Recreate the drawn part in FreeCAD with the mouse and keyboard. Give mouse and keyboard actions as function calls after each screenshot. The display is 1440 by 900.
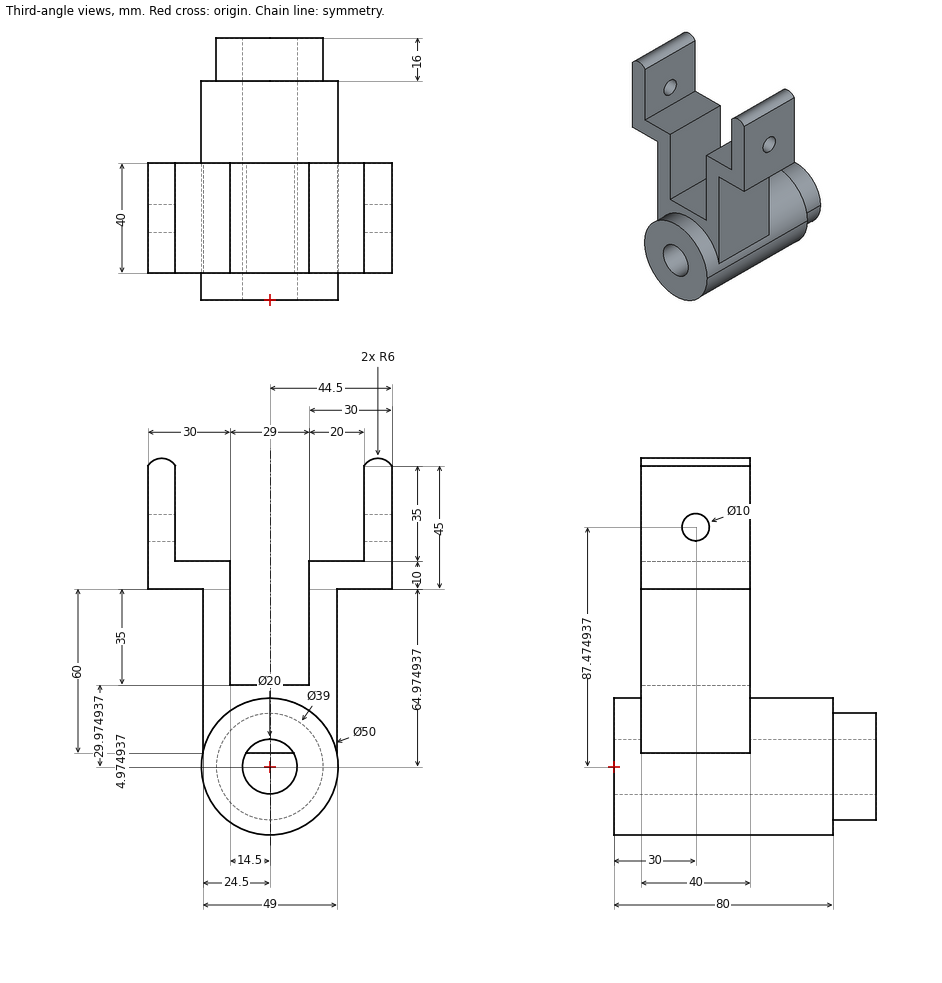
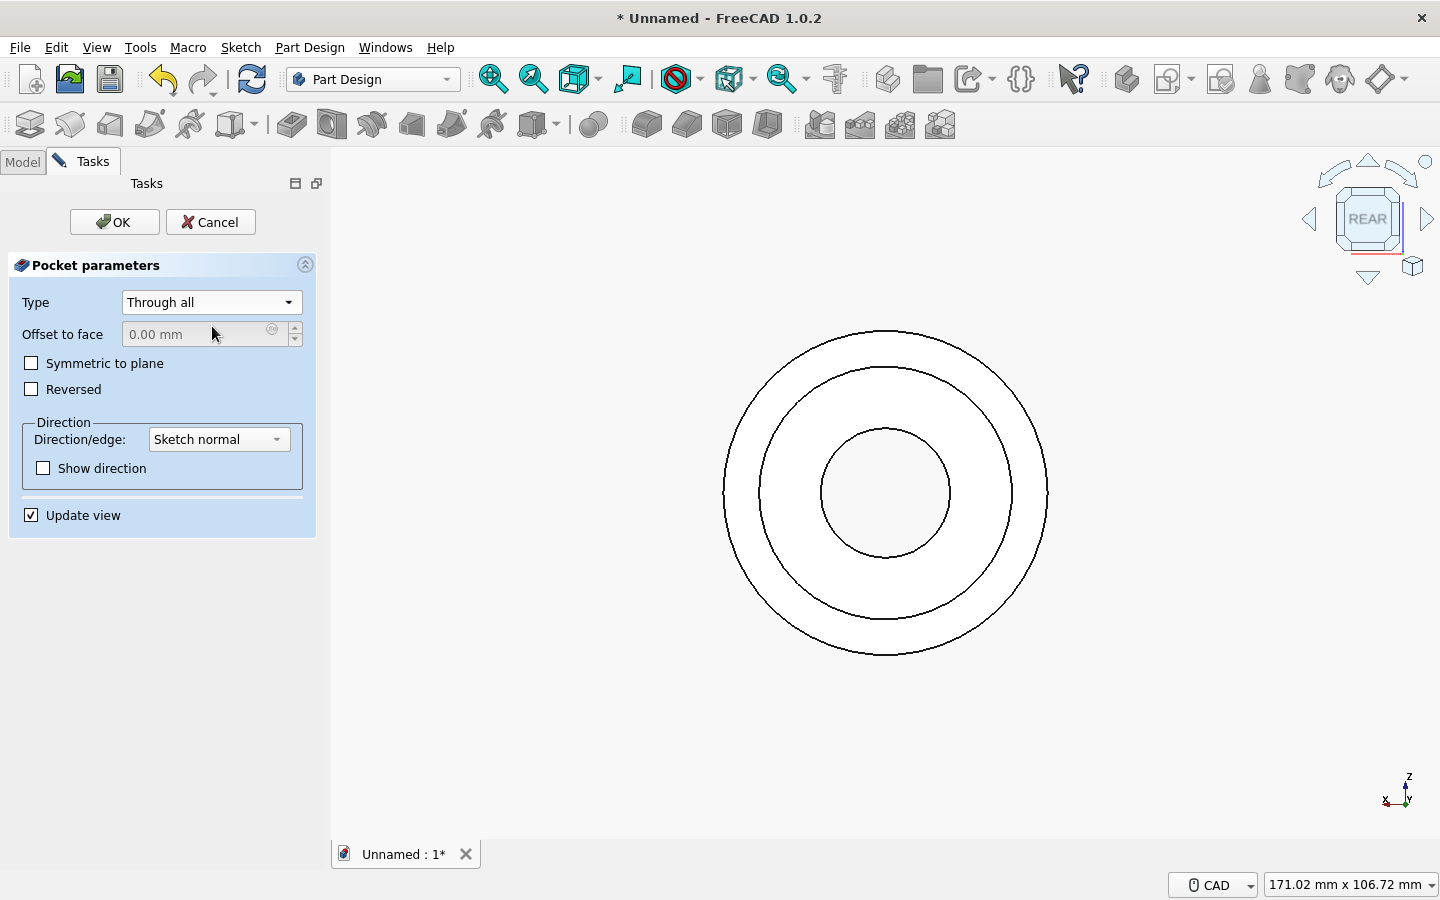
click(115, 222)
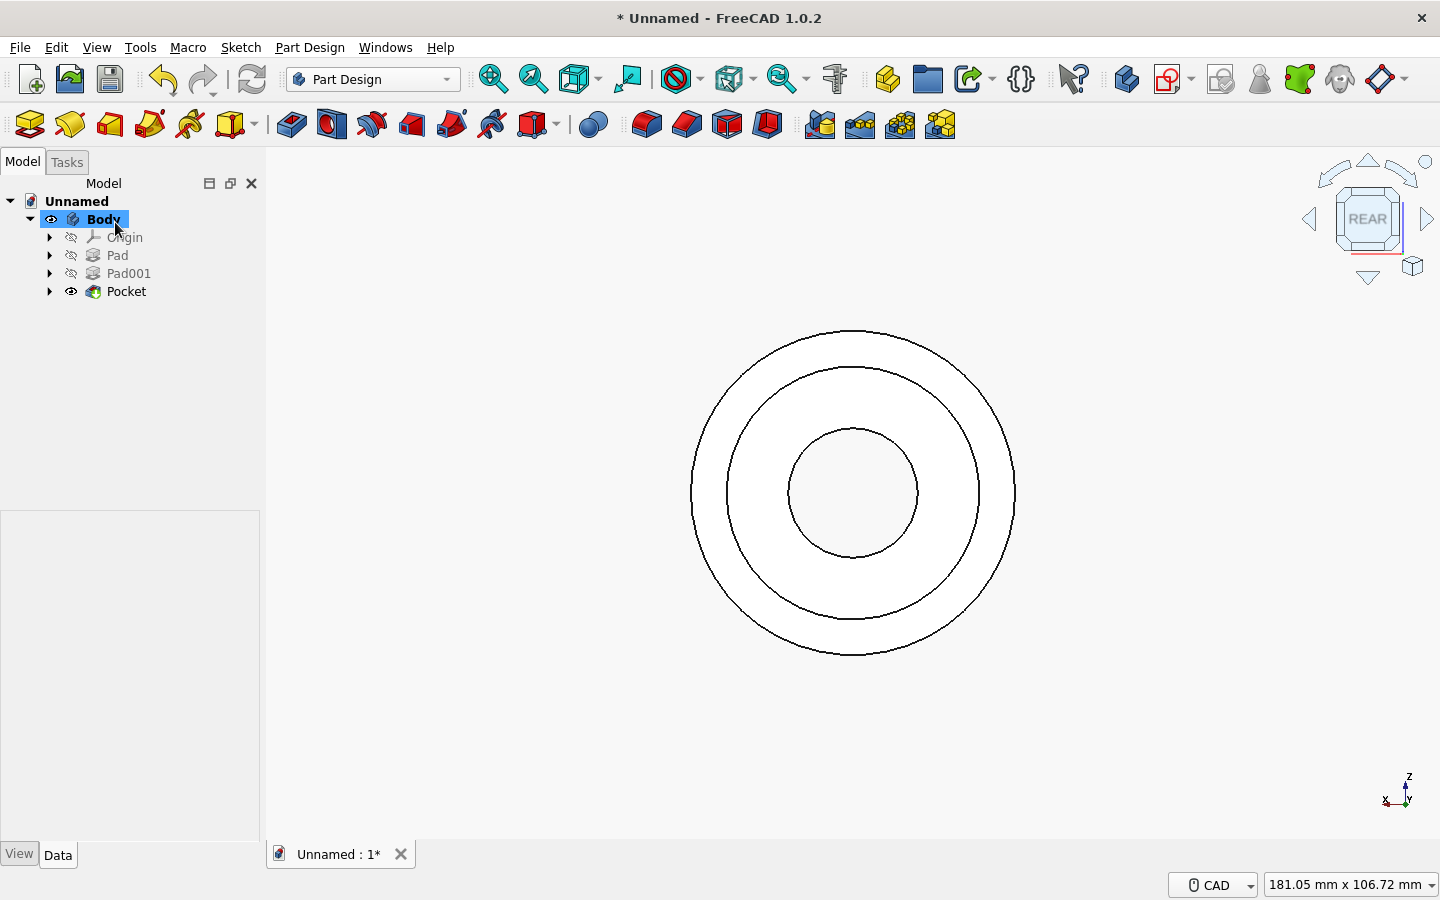
click(50, 237)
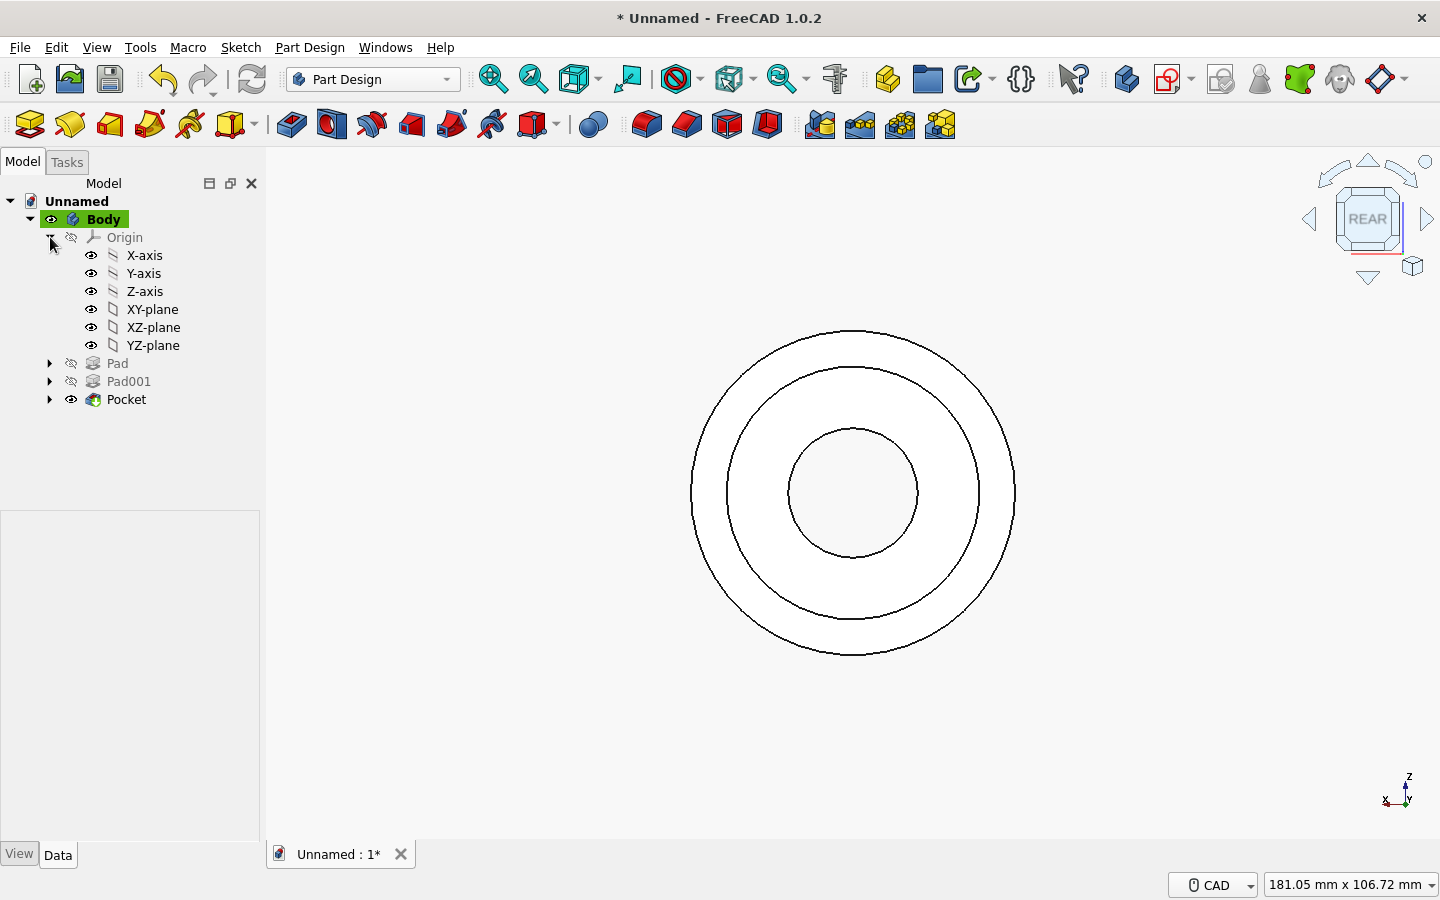
click(136, 327)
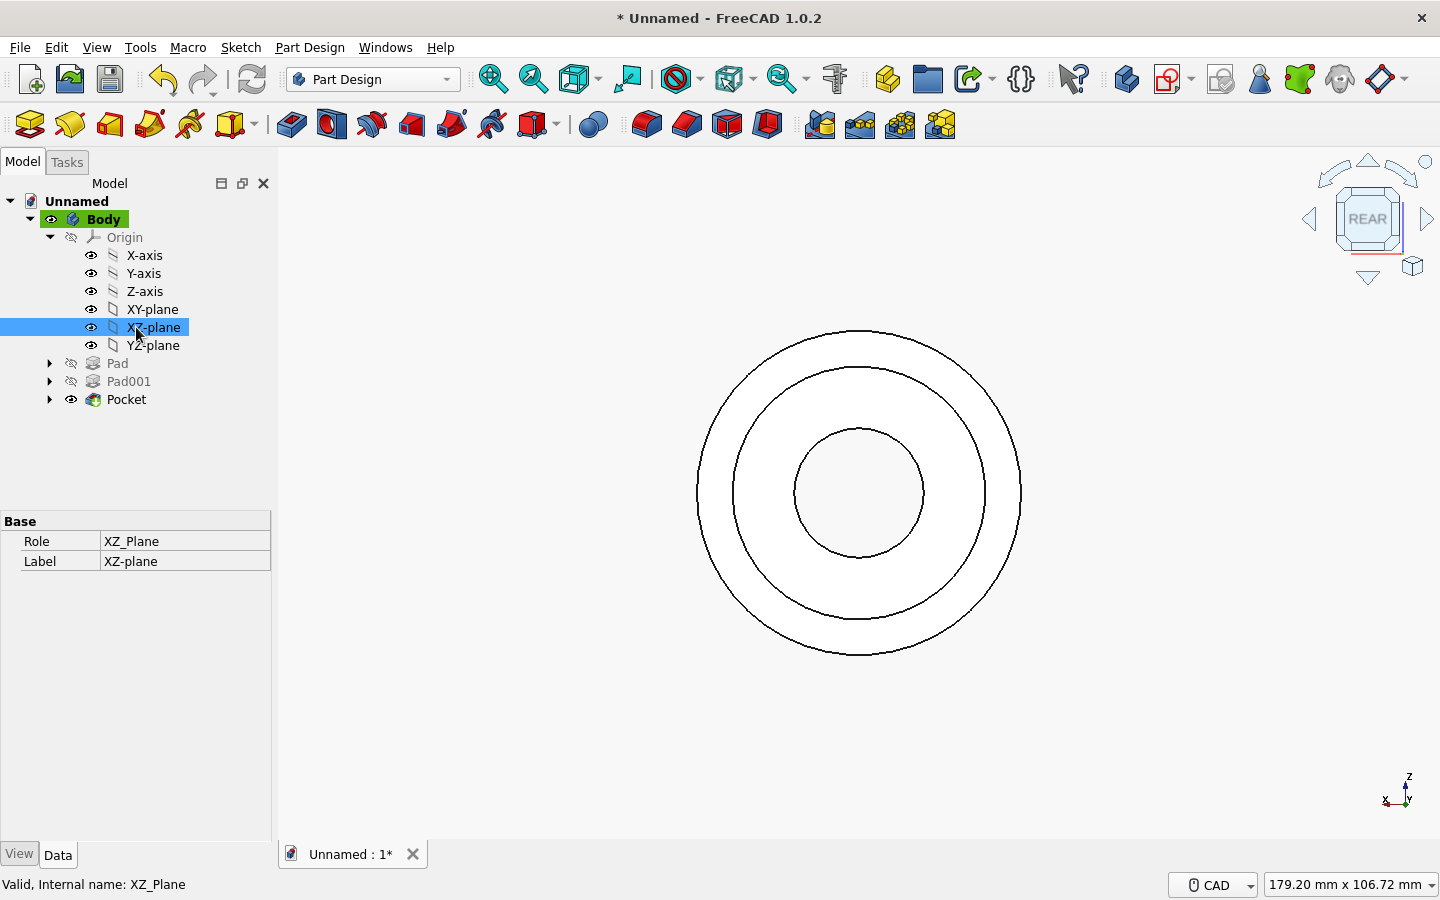
click(1380, 80)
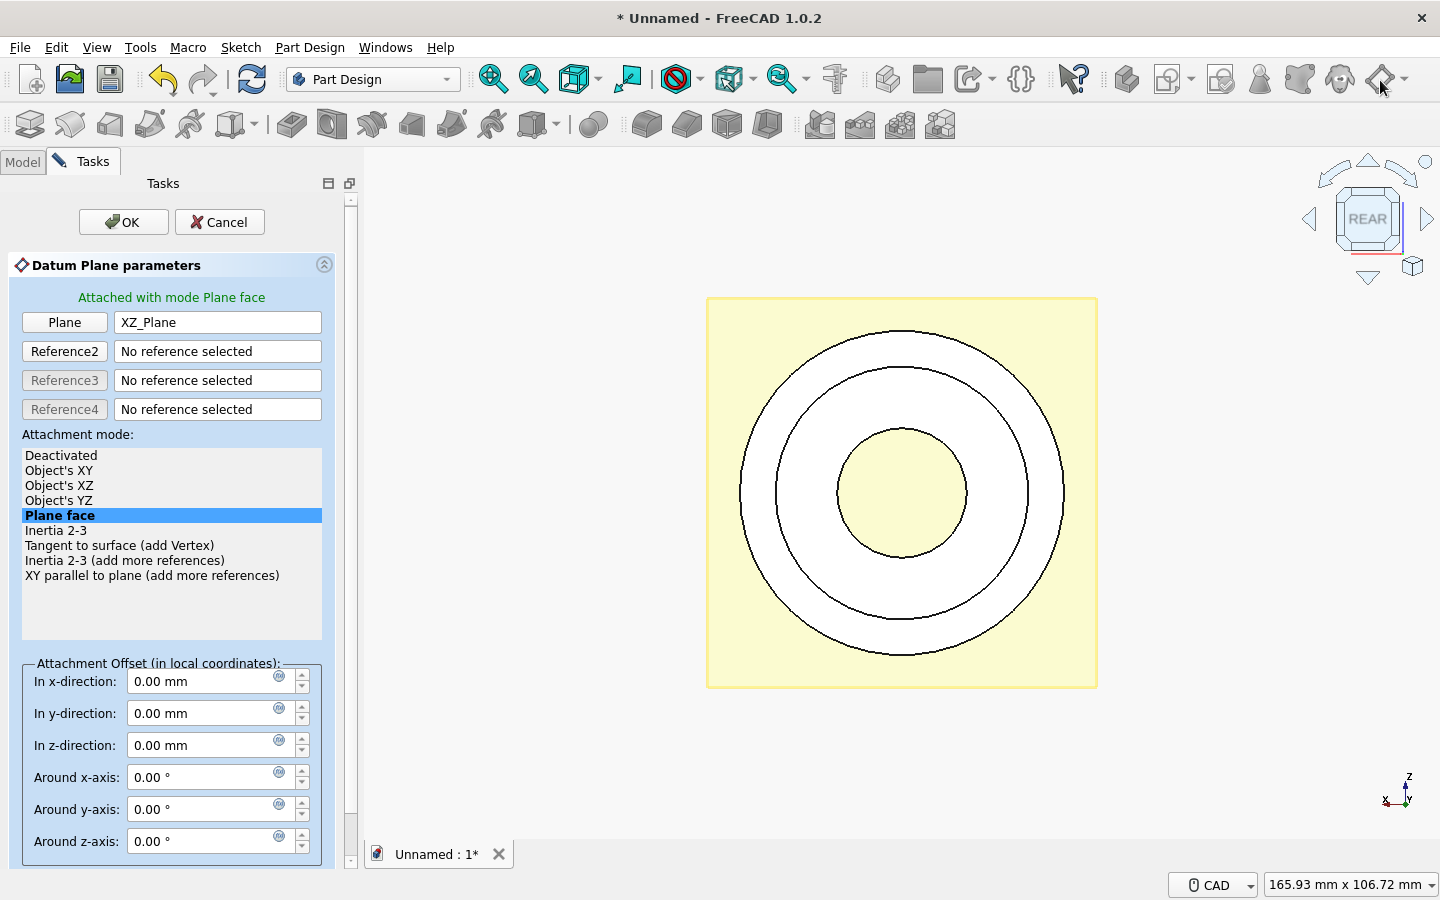
triple_click(210, 745)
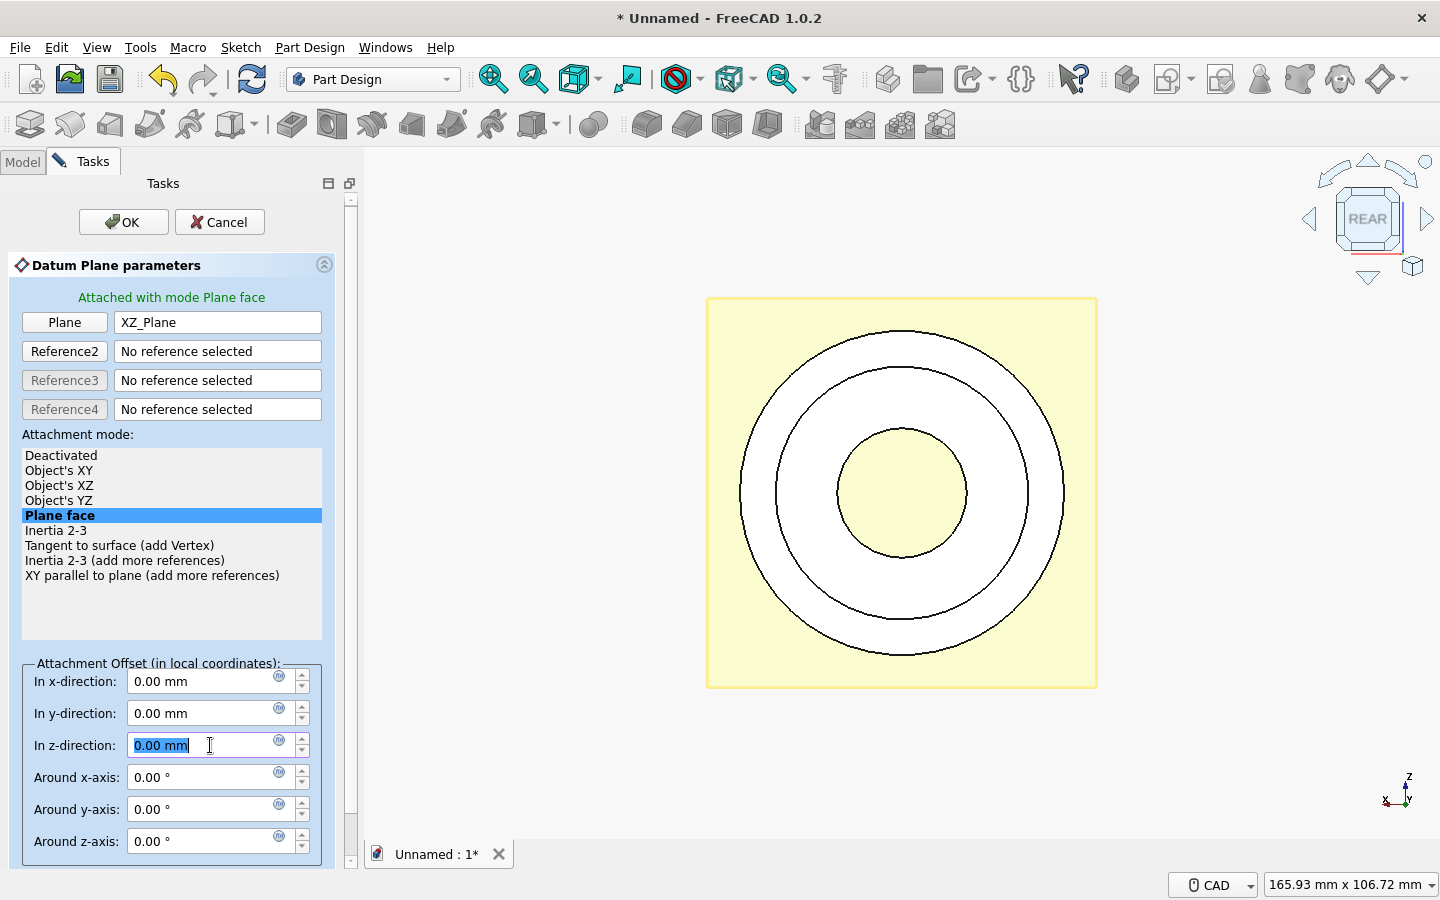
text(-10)
key(Tab)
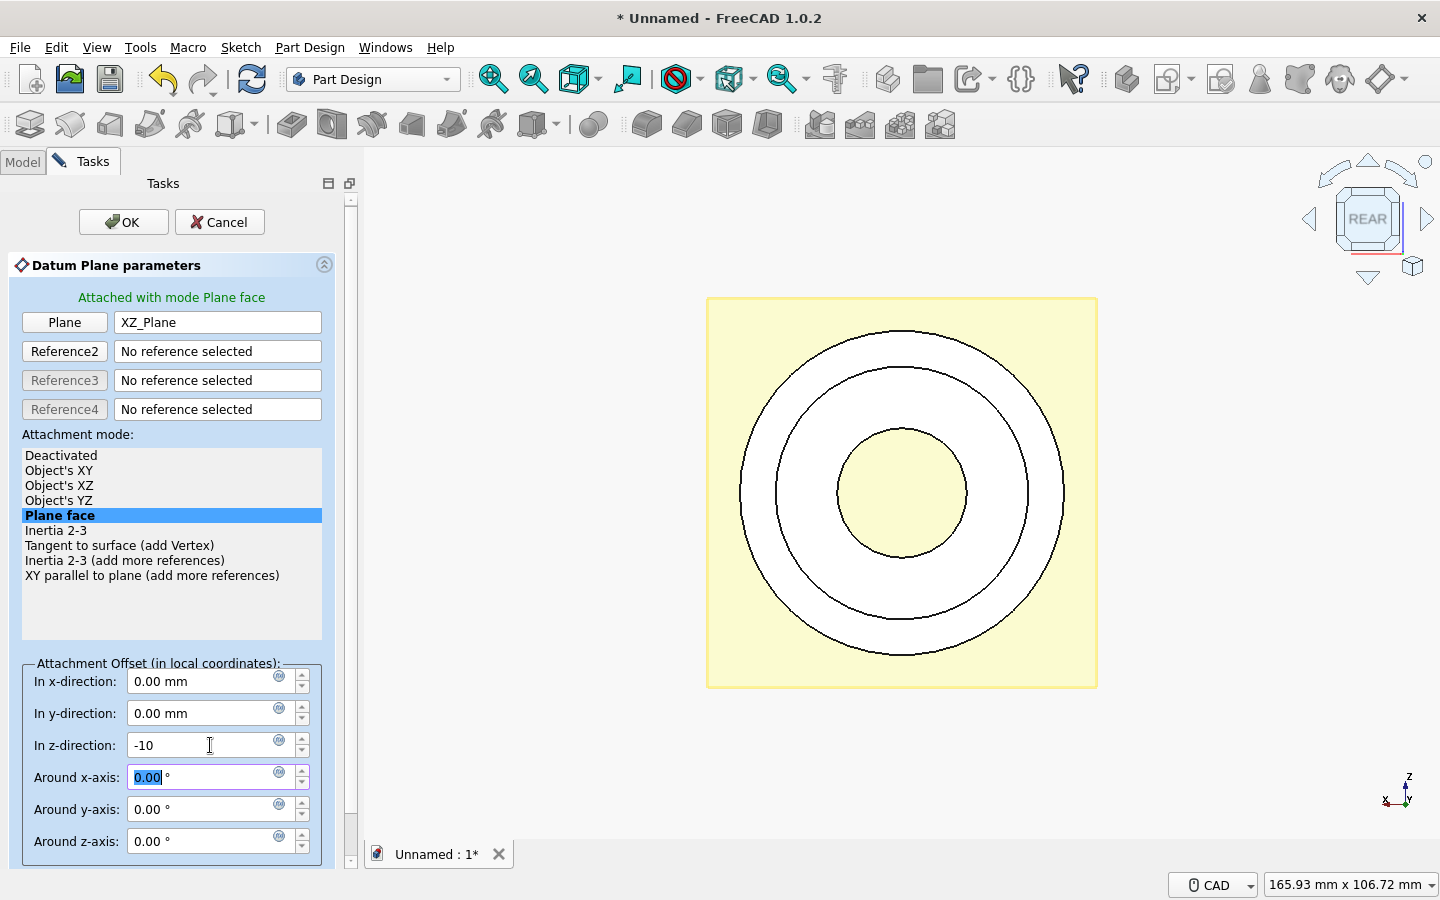
click(124, 222)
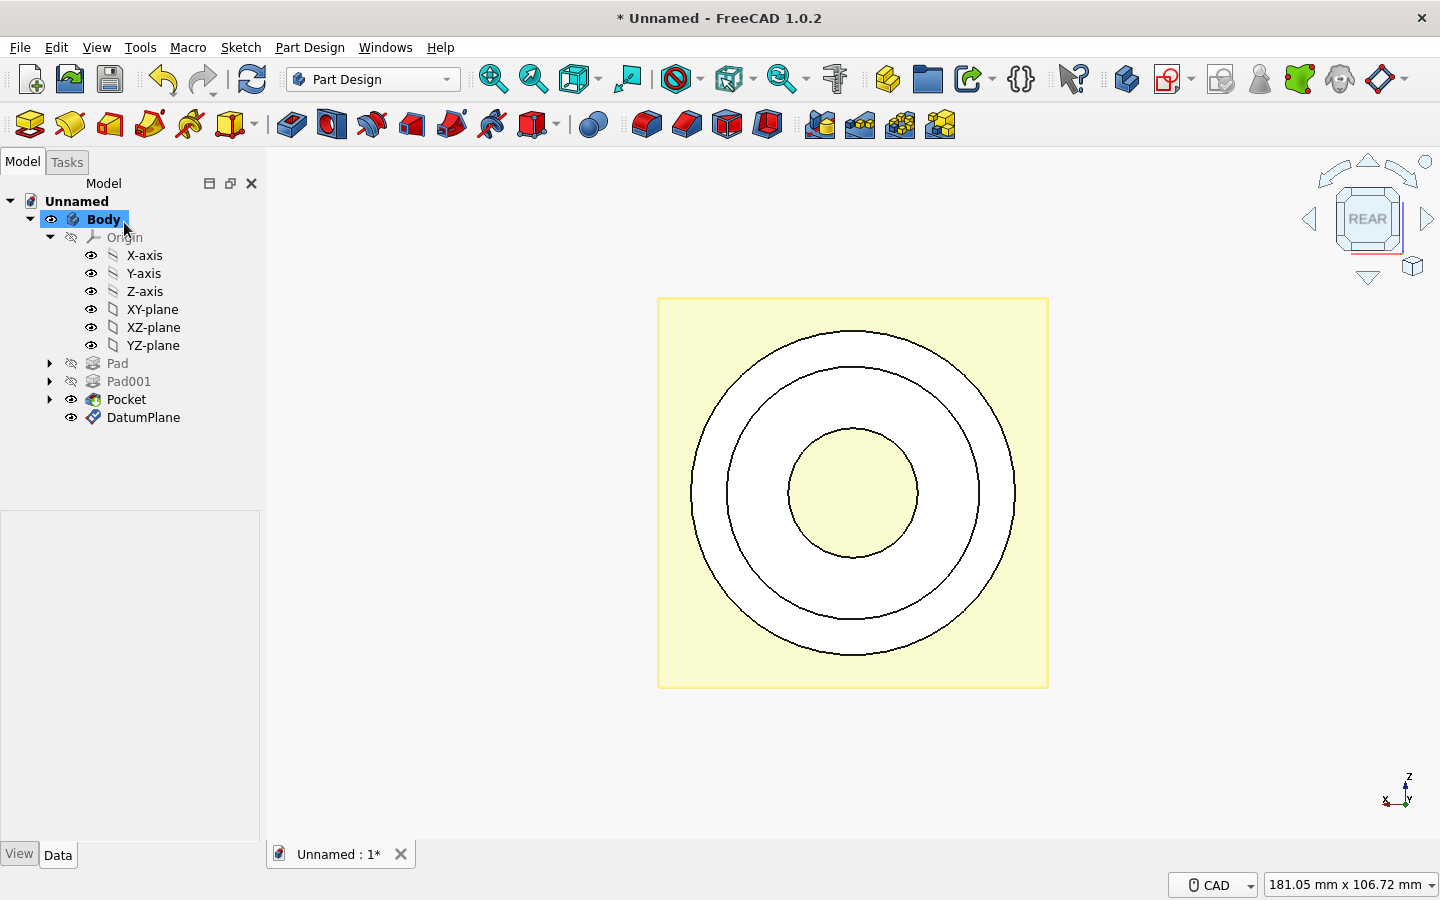
click(116, 417)